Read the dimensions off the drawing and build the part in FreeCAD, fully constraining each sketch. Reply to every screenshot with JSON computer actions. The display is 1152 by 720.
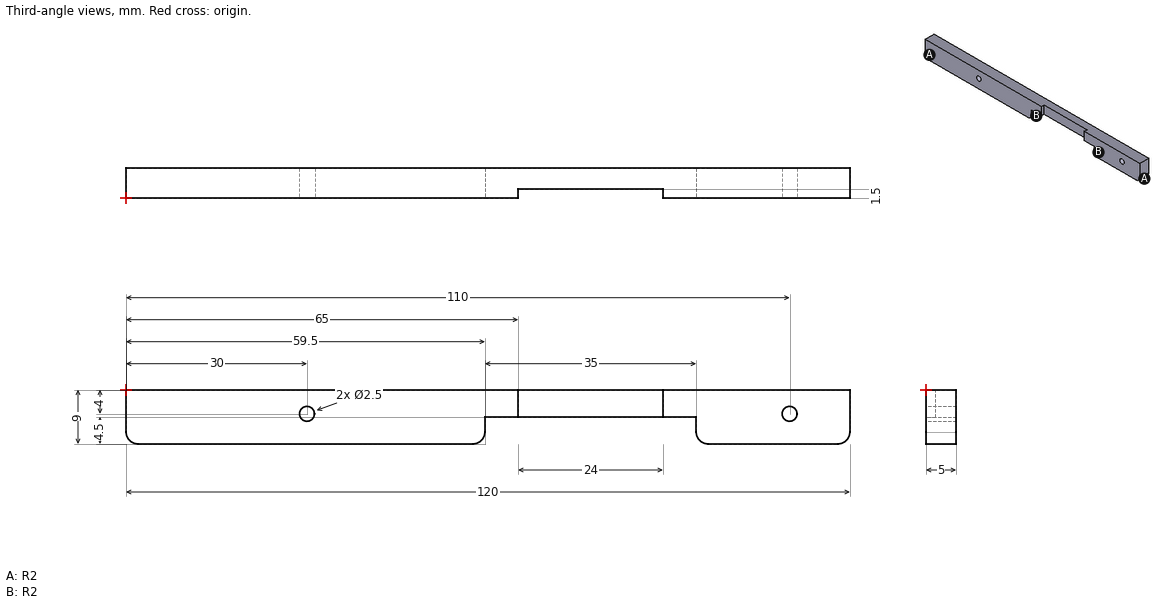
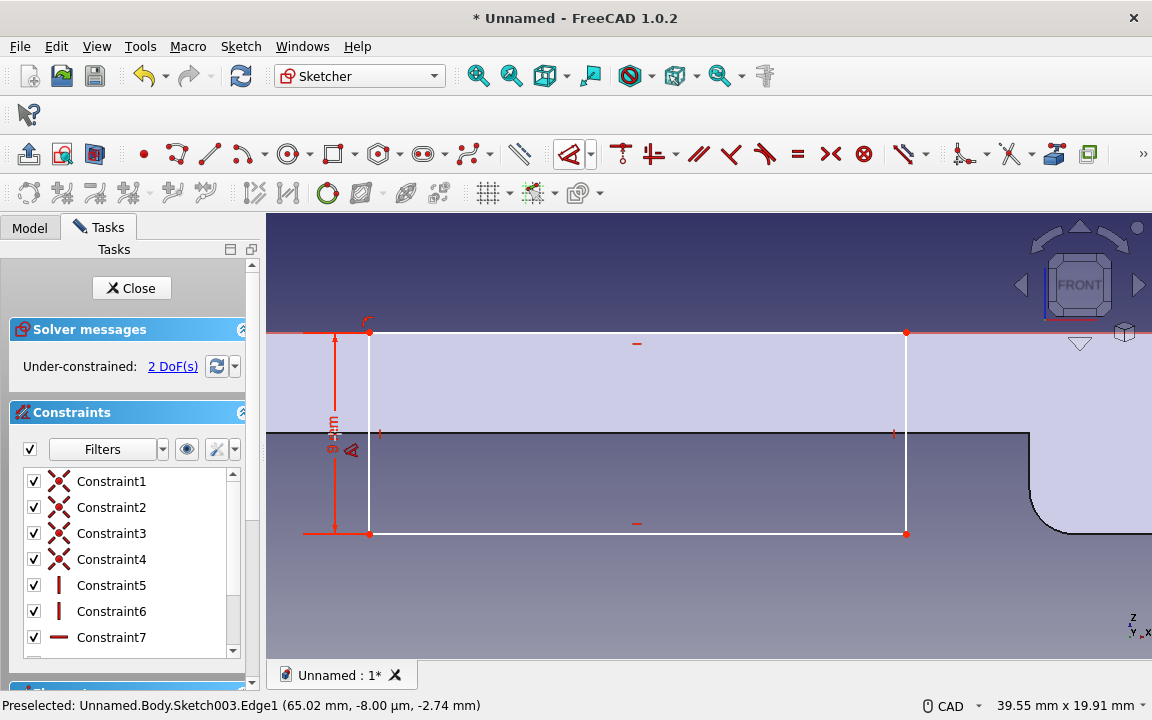
{"action": "left_click", "coordinate": [530, 534]}
{"action": "left_click", "coordinate": [637, 568]}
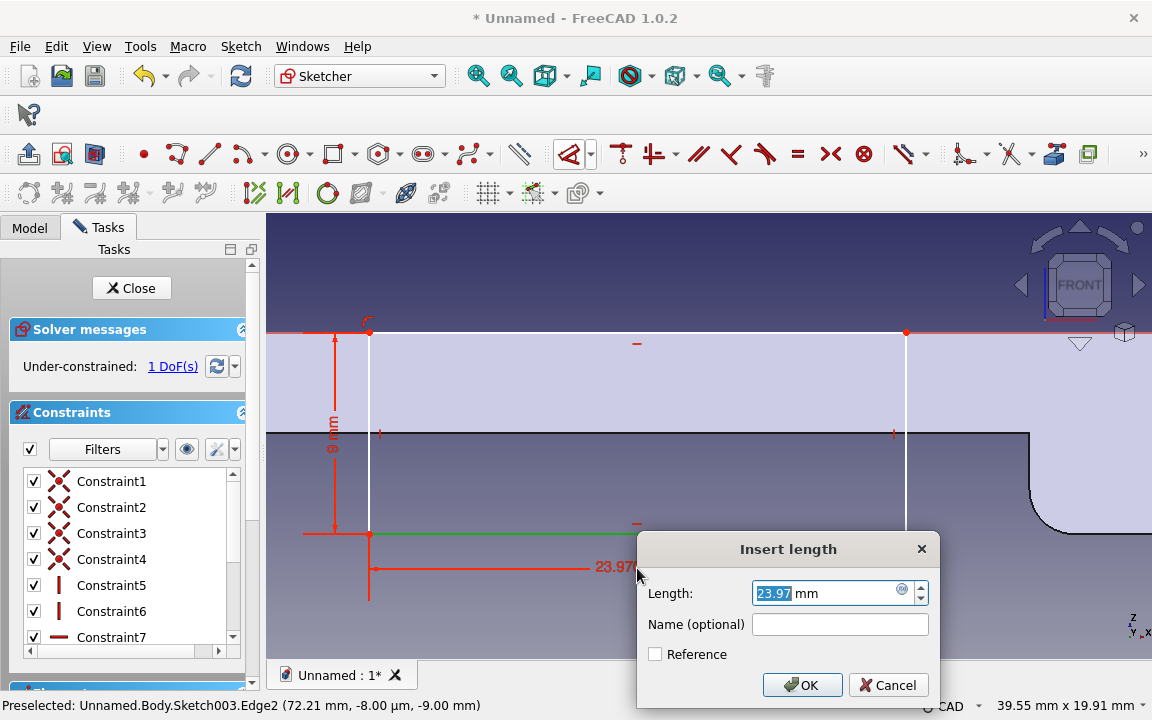
{"action": "type", "text": "24"}
{"action": "key", "text": "Return"}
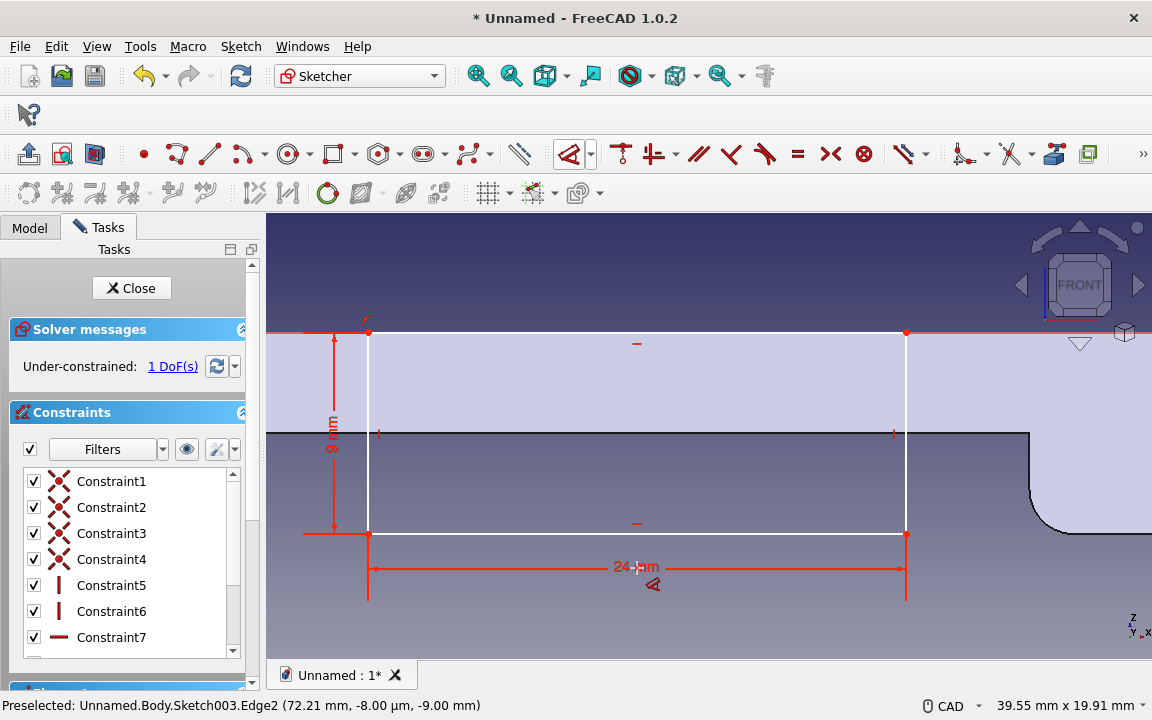
{"action": "left_click", "coordinate": [368, 333]}
{"action": "left_click", "coordinate": [331, 299]}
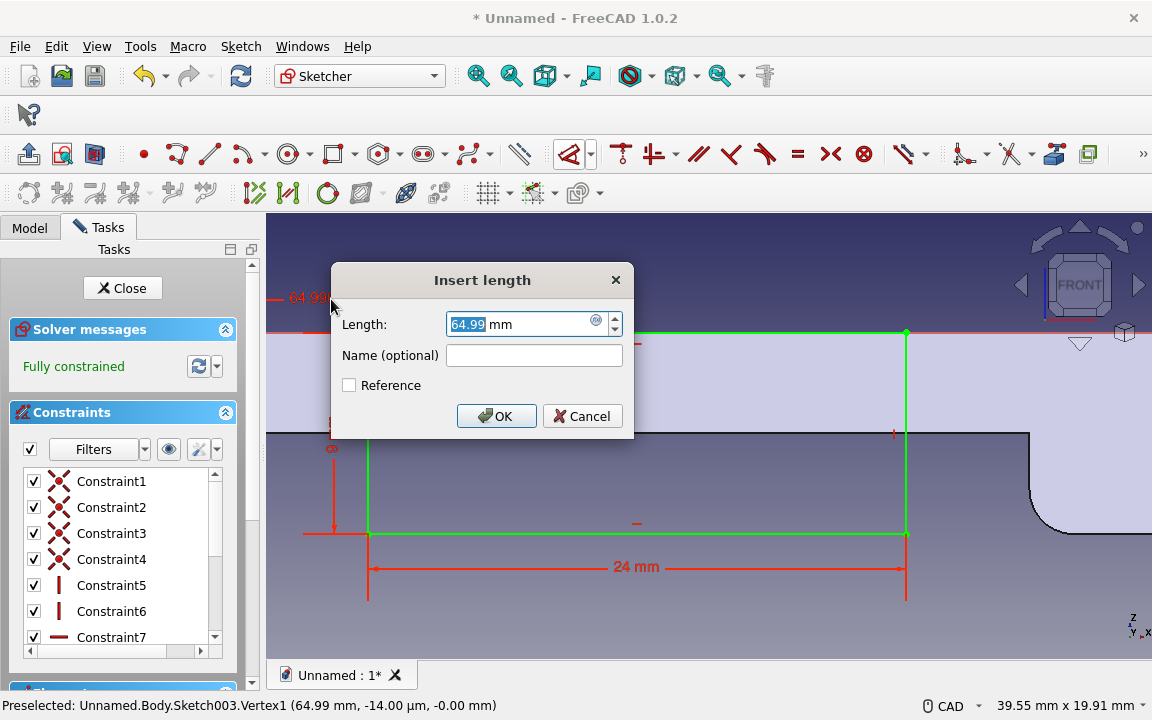
{"action": "type", "text": "65"}
{"action": "key", "text": "Return"}
{"action": "key", "text": "Escape"}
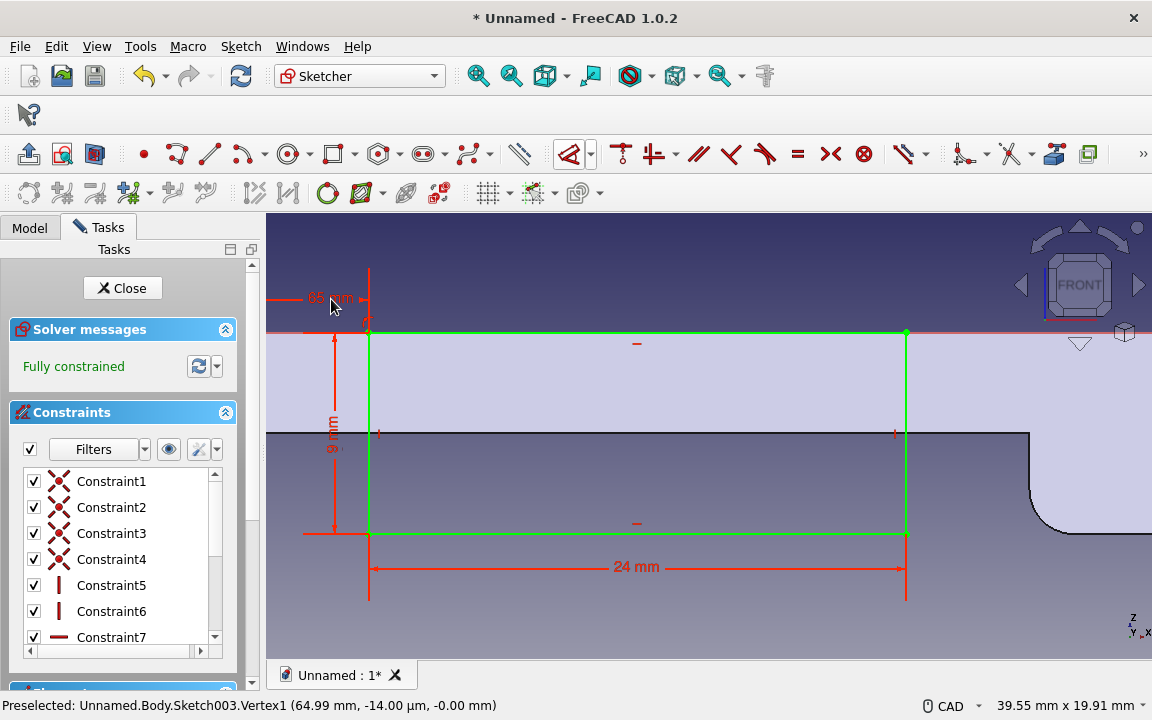
{"action": "left_click", "coordinate": [123, 288]}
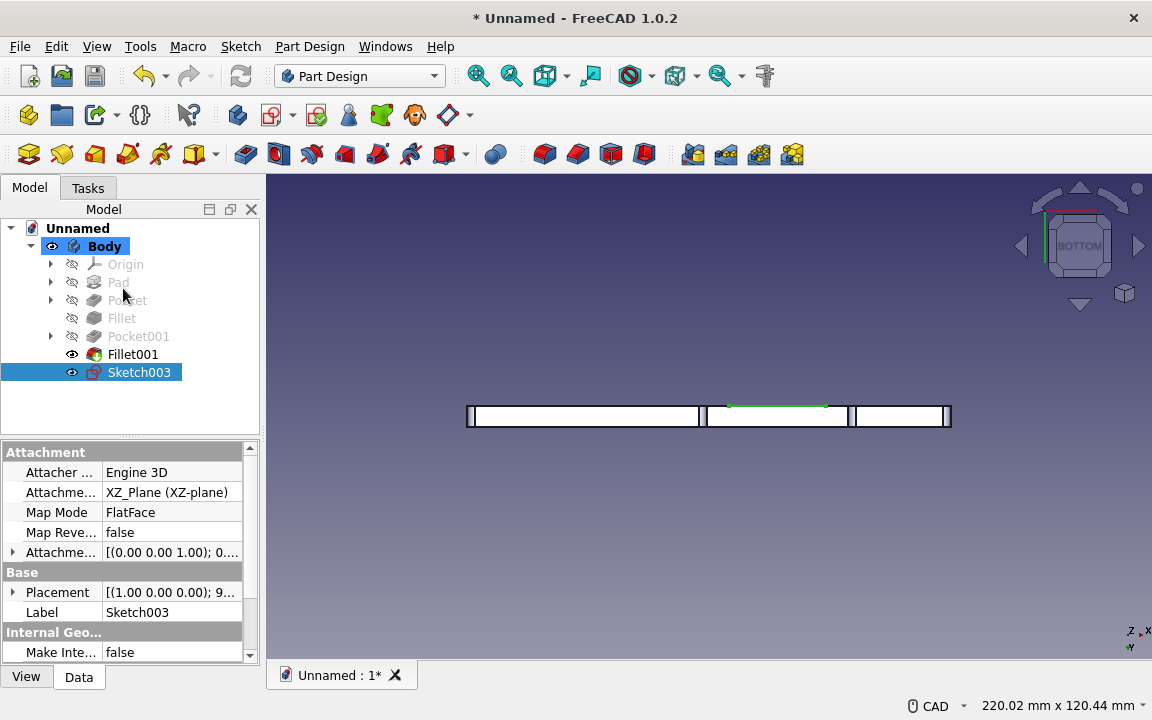
{"action": "left_click", "coordinate": [246, 154]}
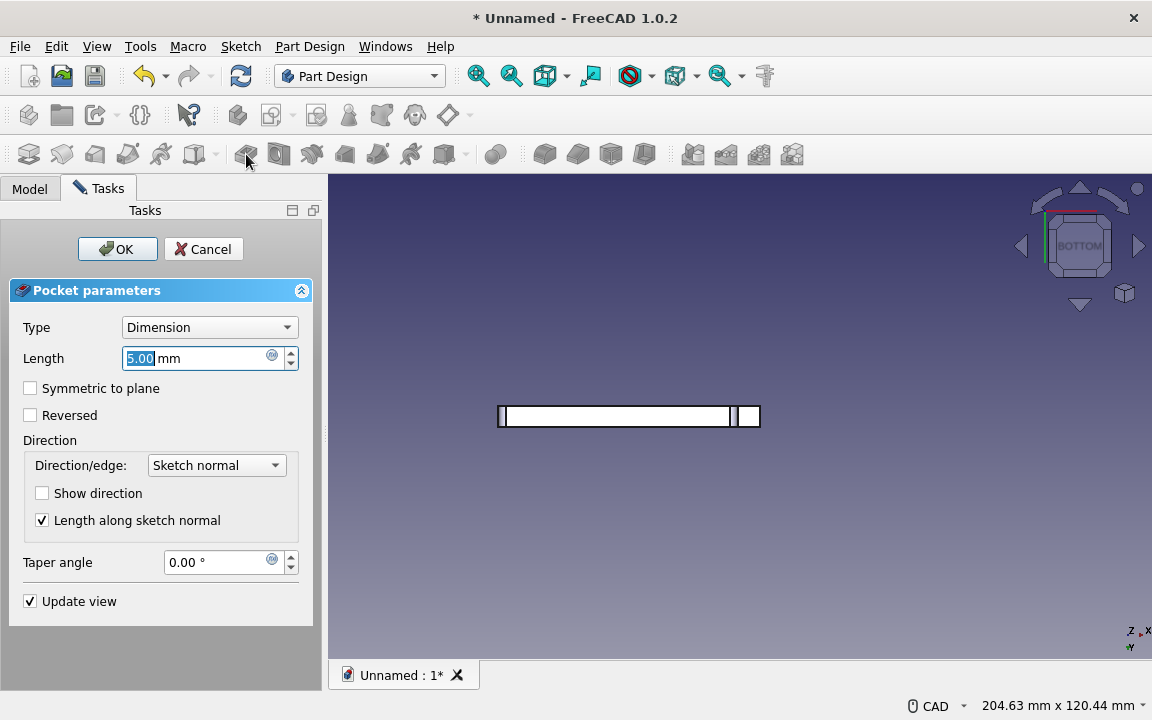
{"action": "type", "text": "1.5"}
{"action": "key", "text": "Tab"}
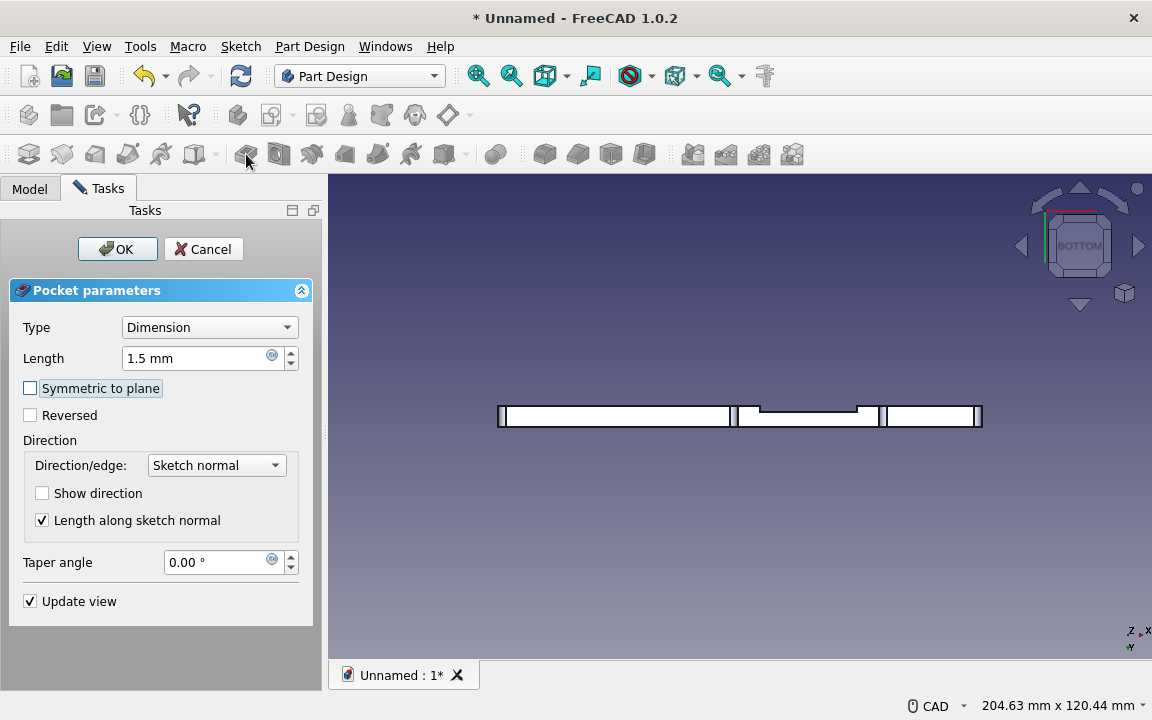
{"action": "left_click", "coordinate": [118, 249]}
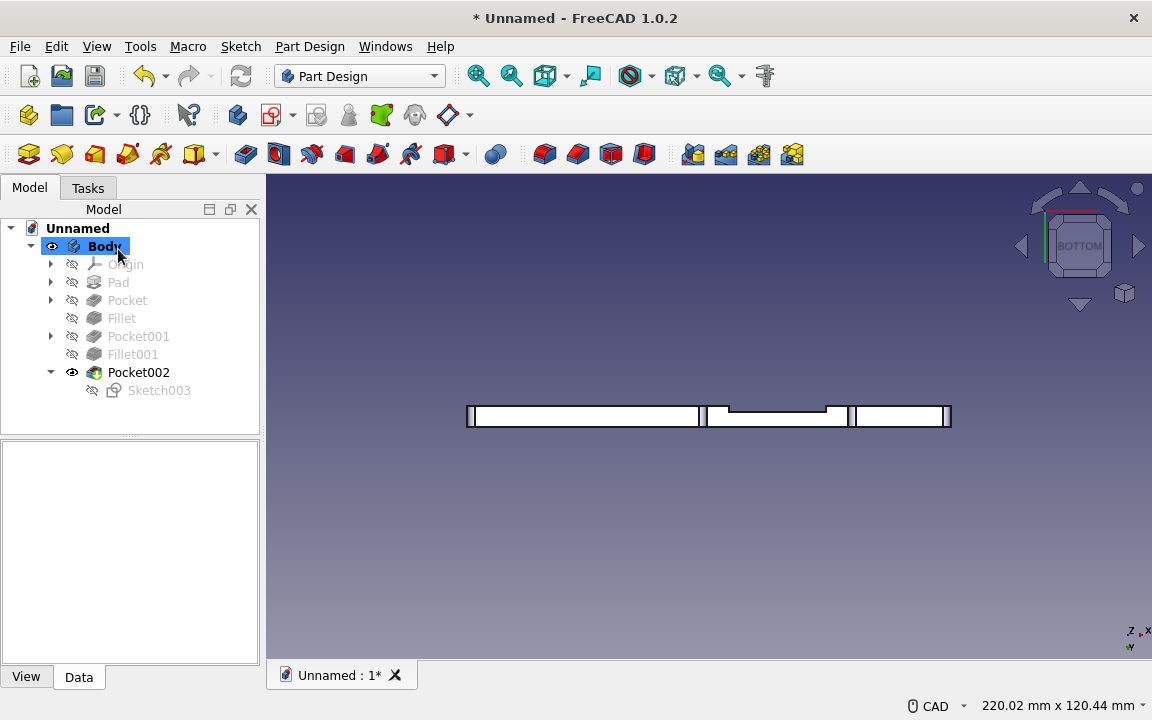
{"action": "key", "text": "0"}